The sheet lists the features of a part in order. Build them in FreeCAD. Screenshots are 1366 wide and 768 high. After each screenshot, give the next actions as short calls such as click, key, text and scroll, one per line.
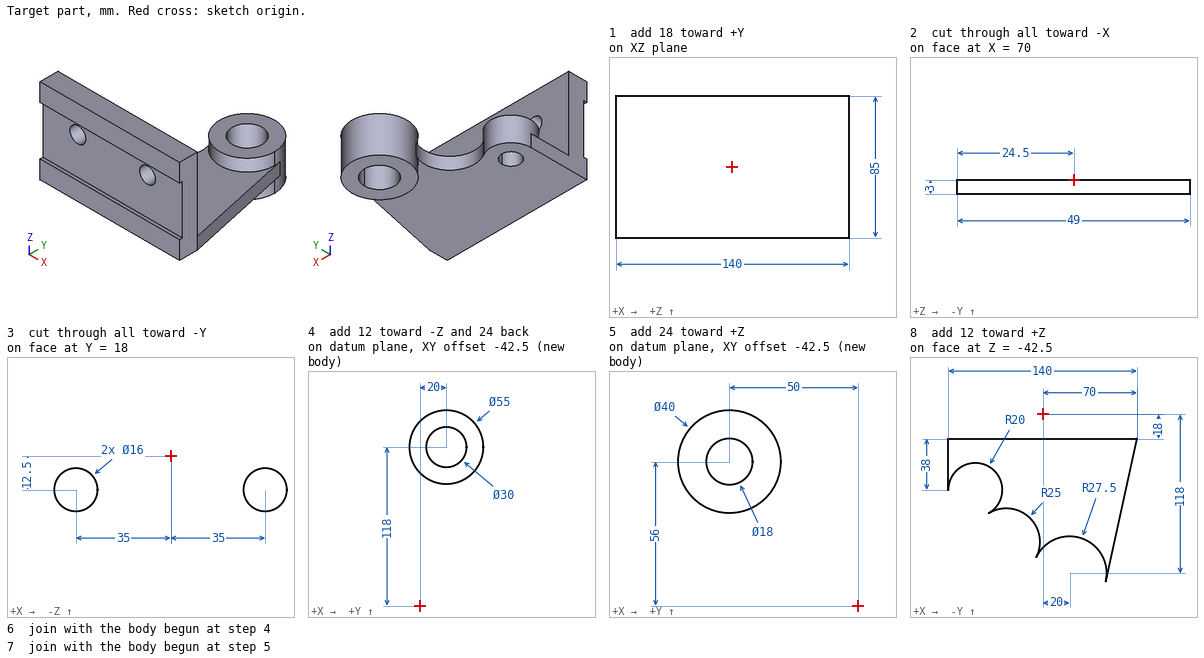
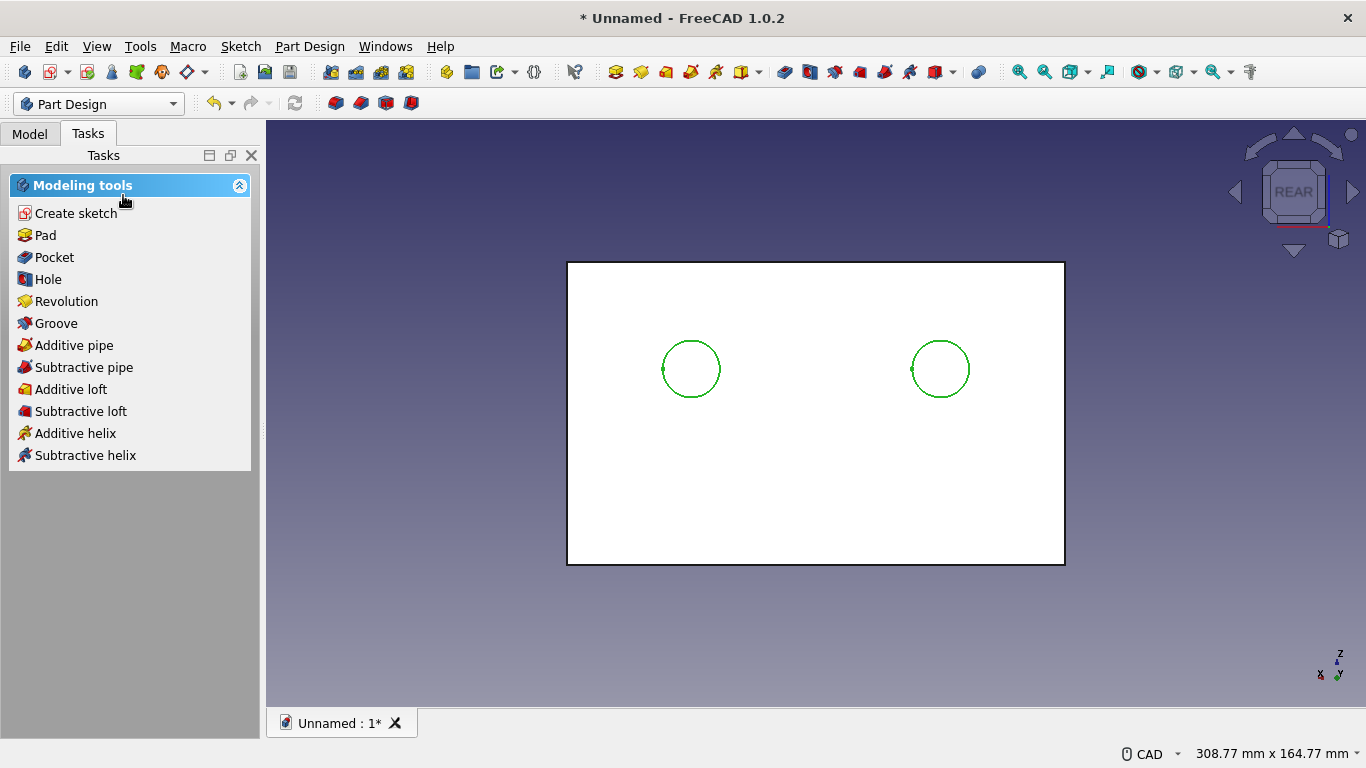
click(785, 72)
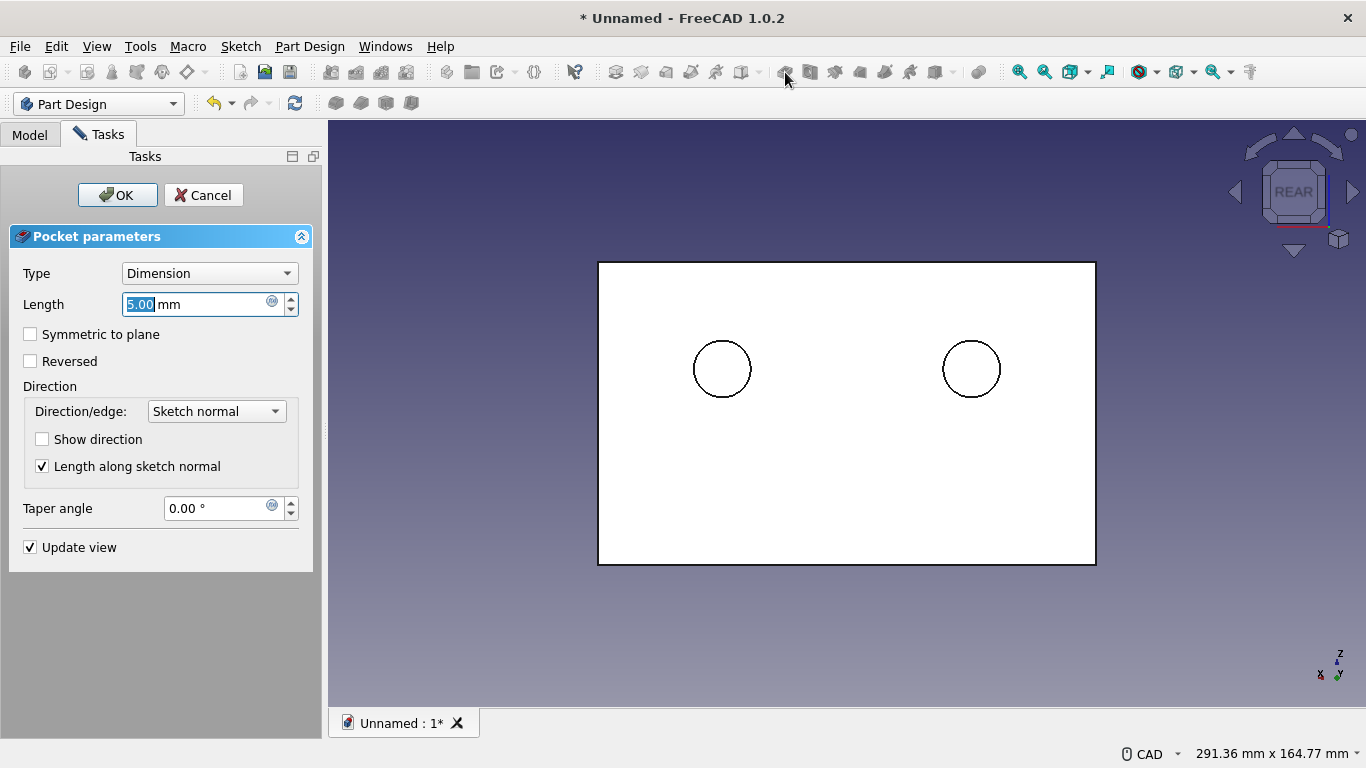
click(210, 274)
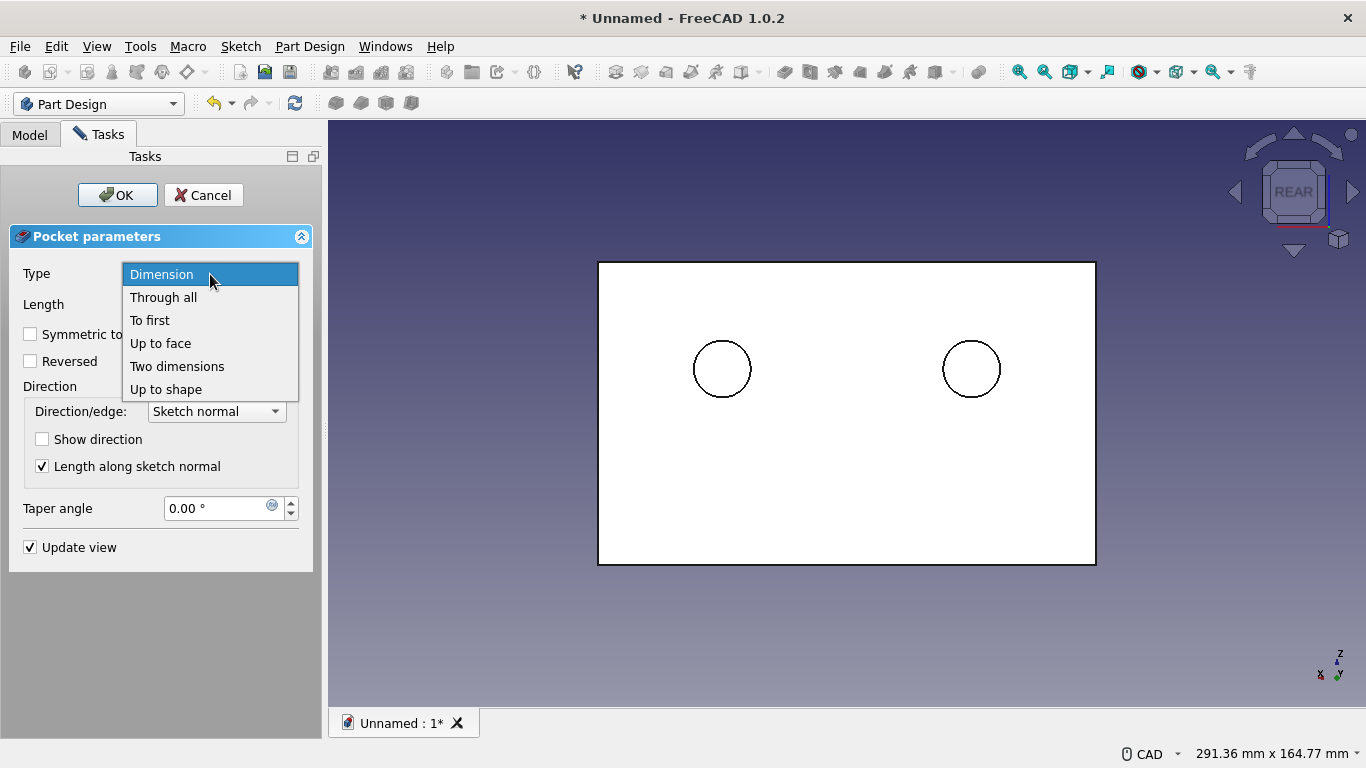
click(208, 298)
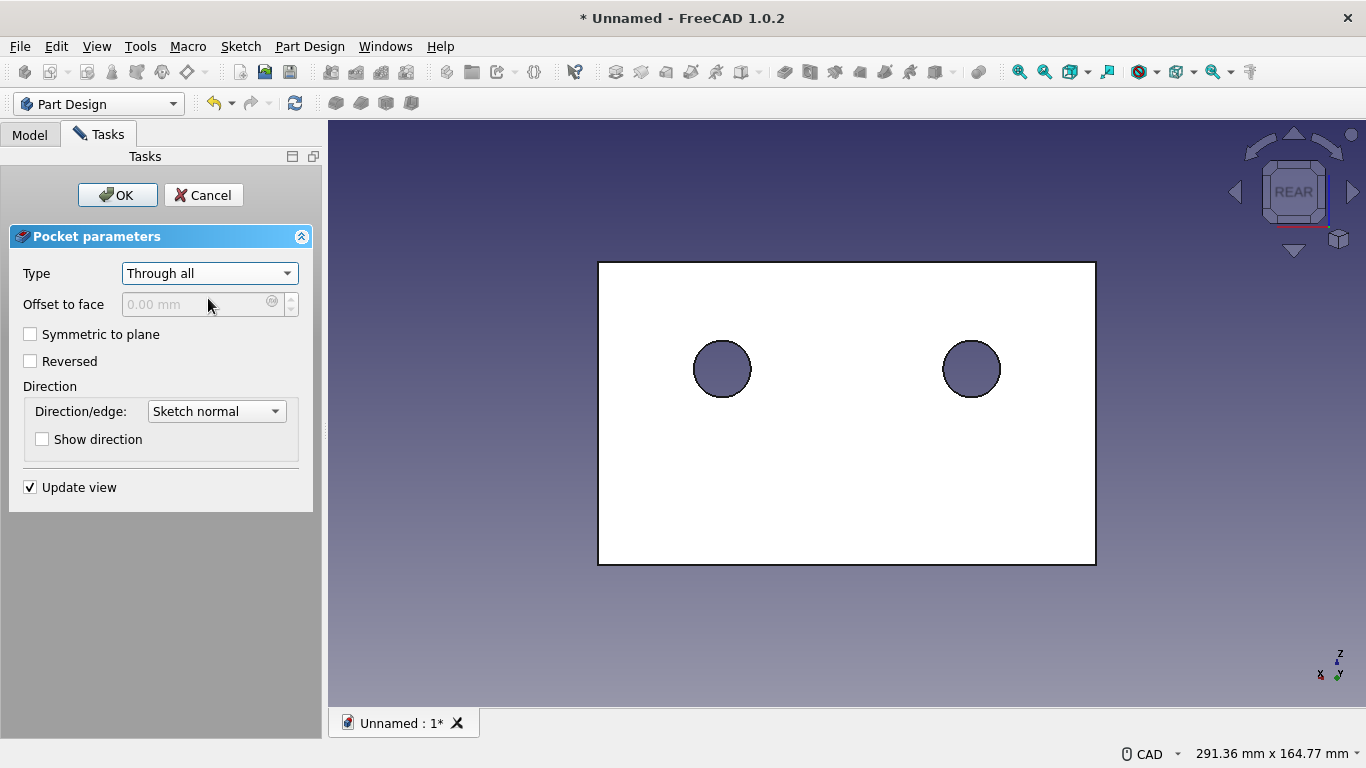
click(118, 195)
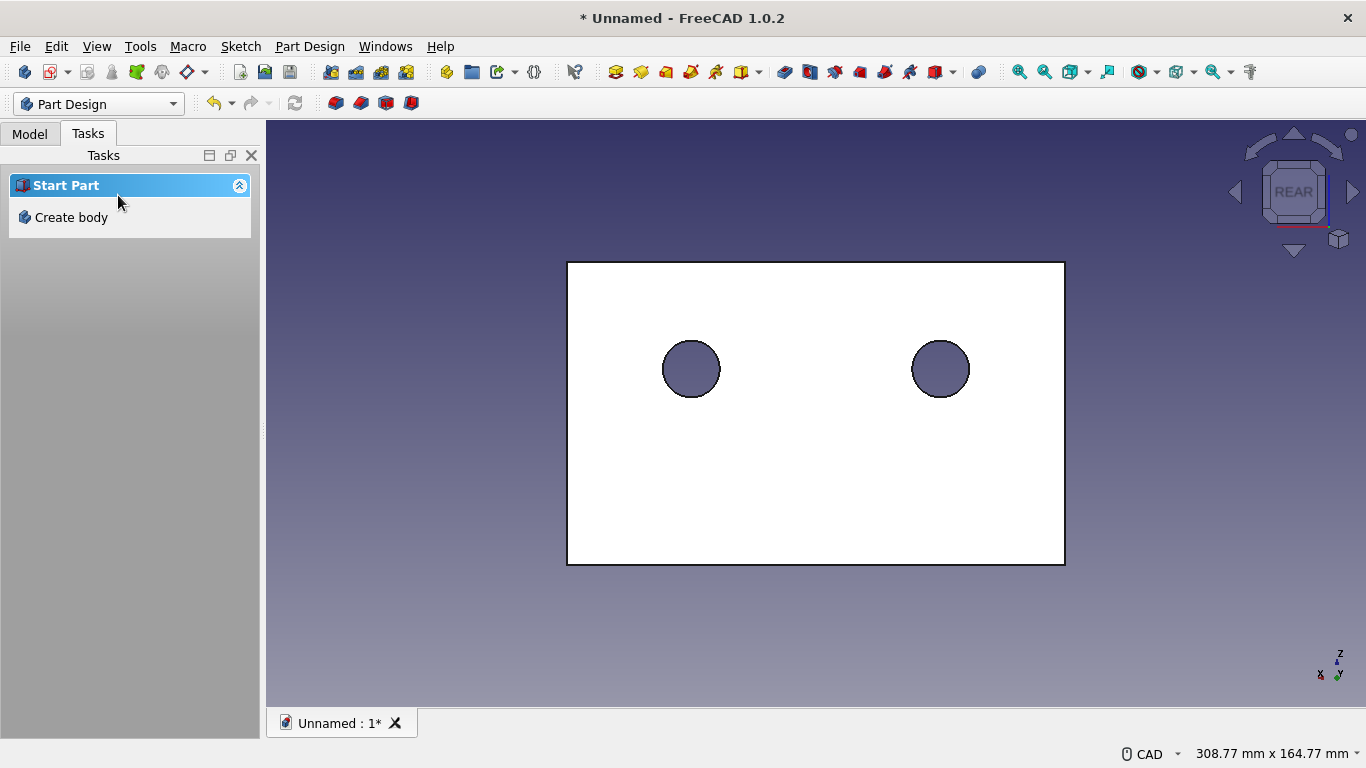
click(25, 72)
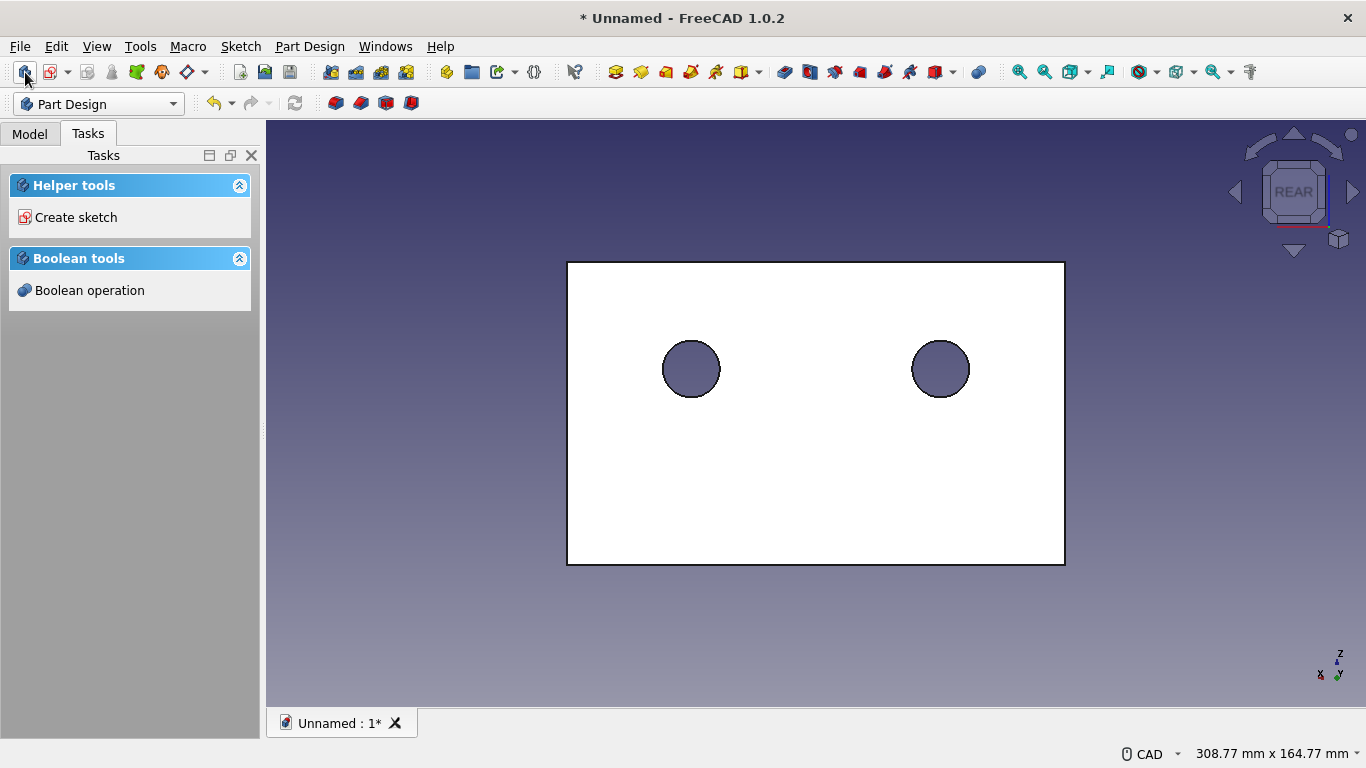
click(30, 134)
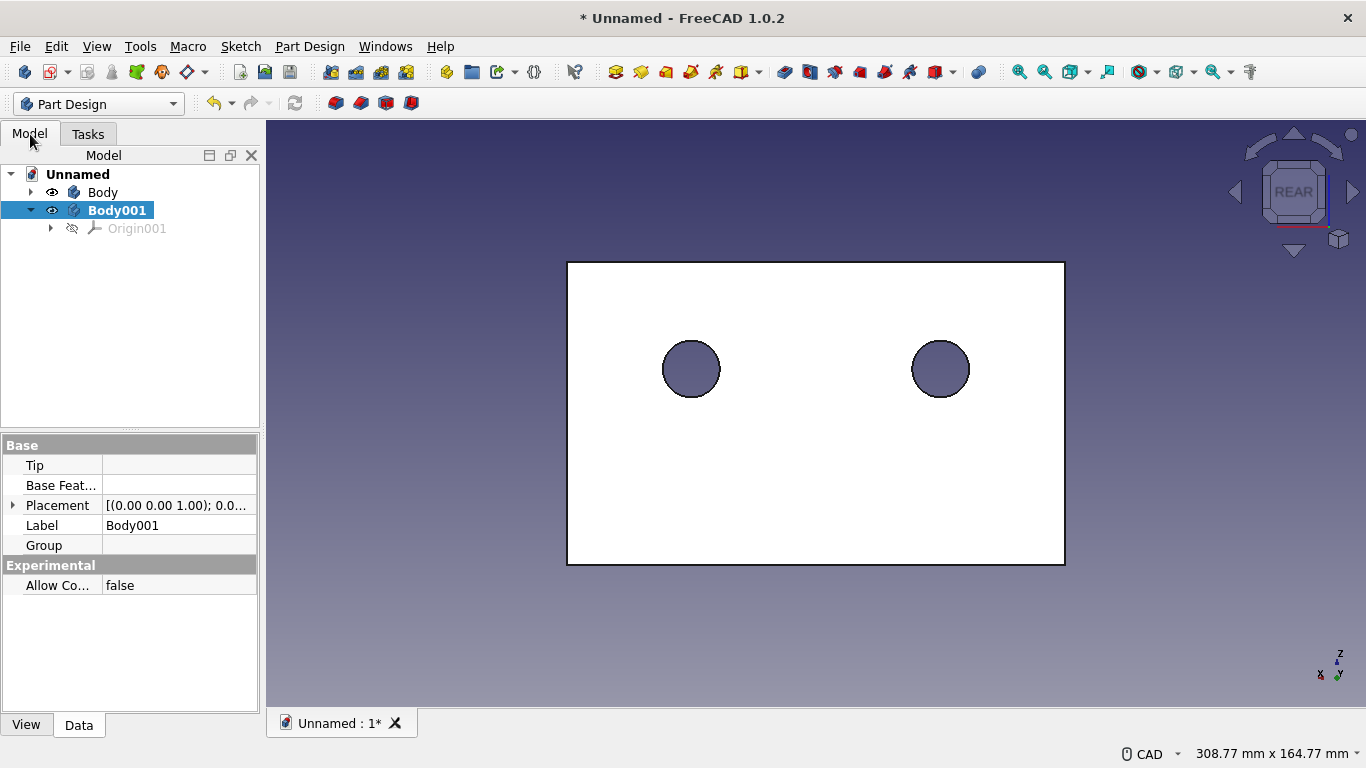
click(51, 228)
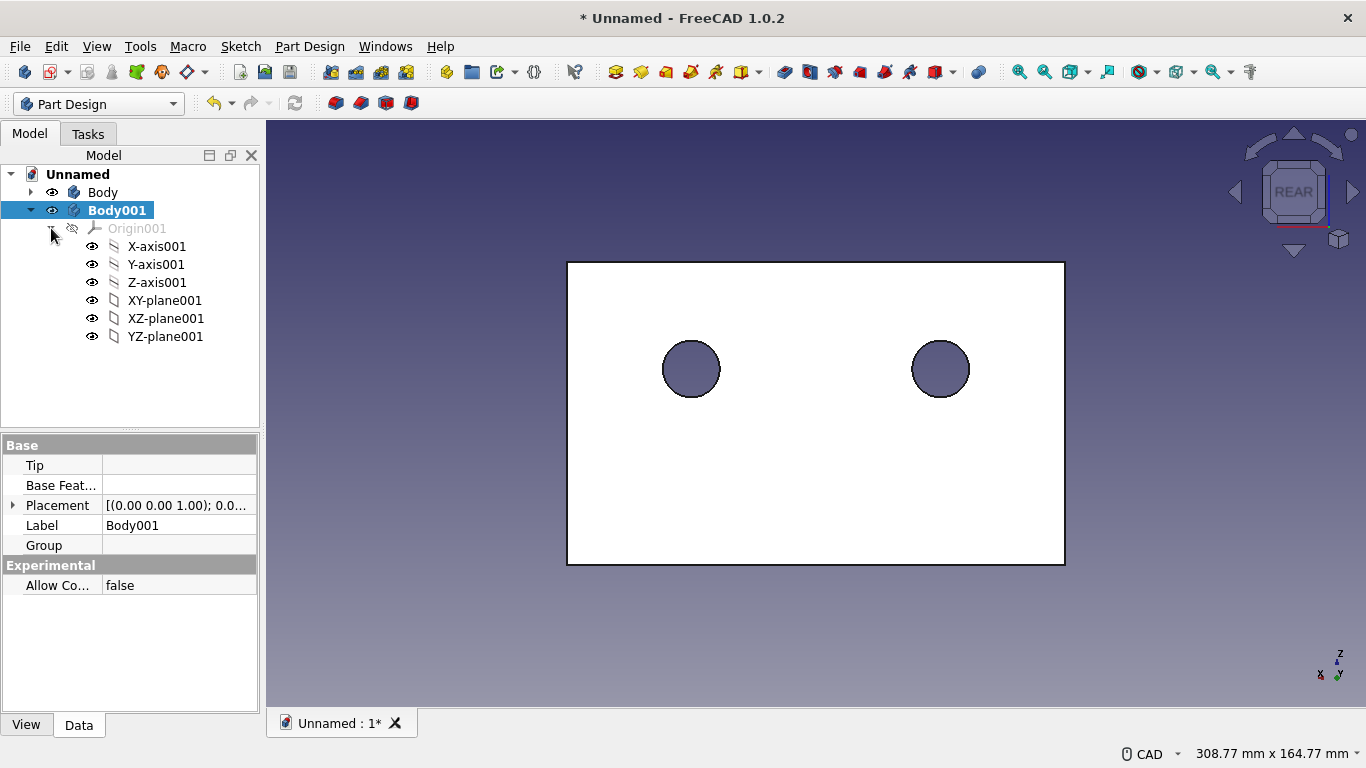
click(137, 300)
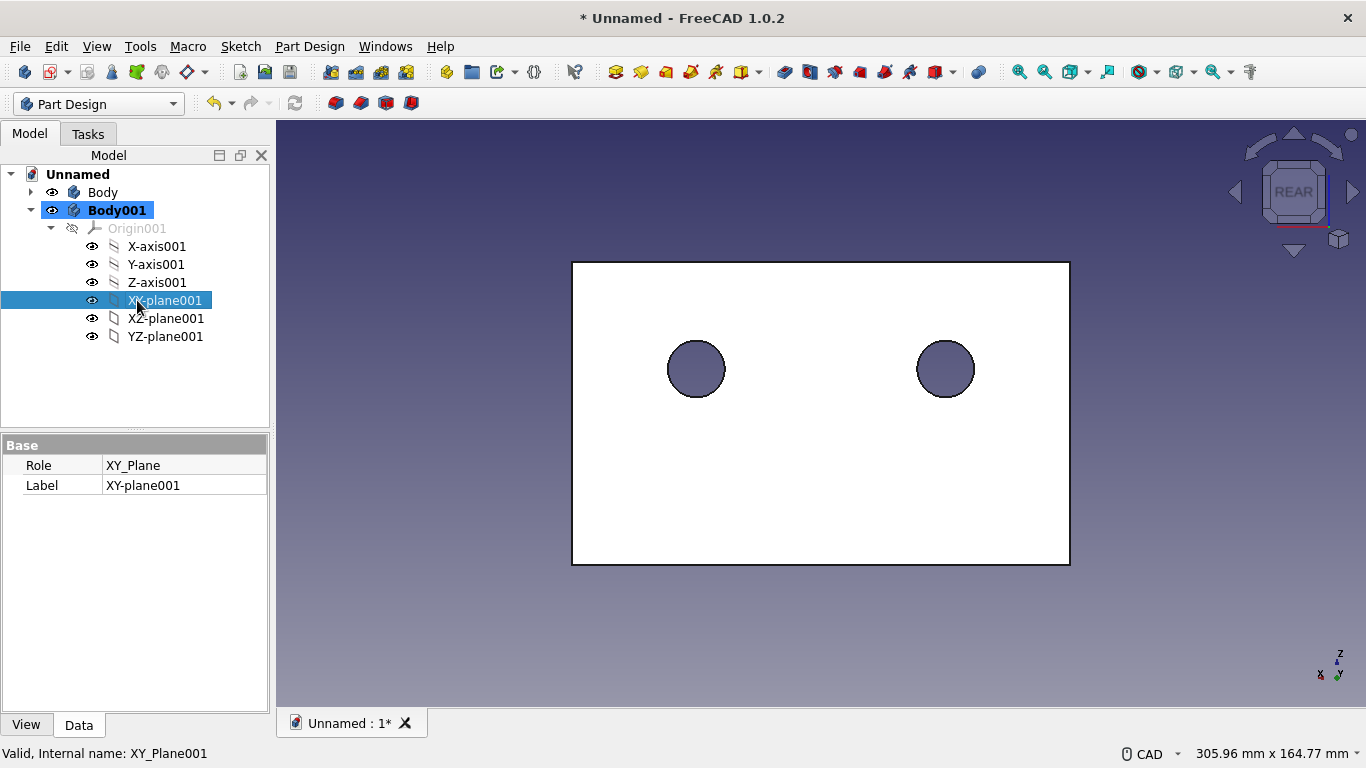
click(186, 72)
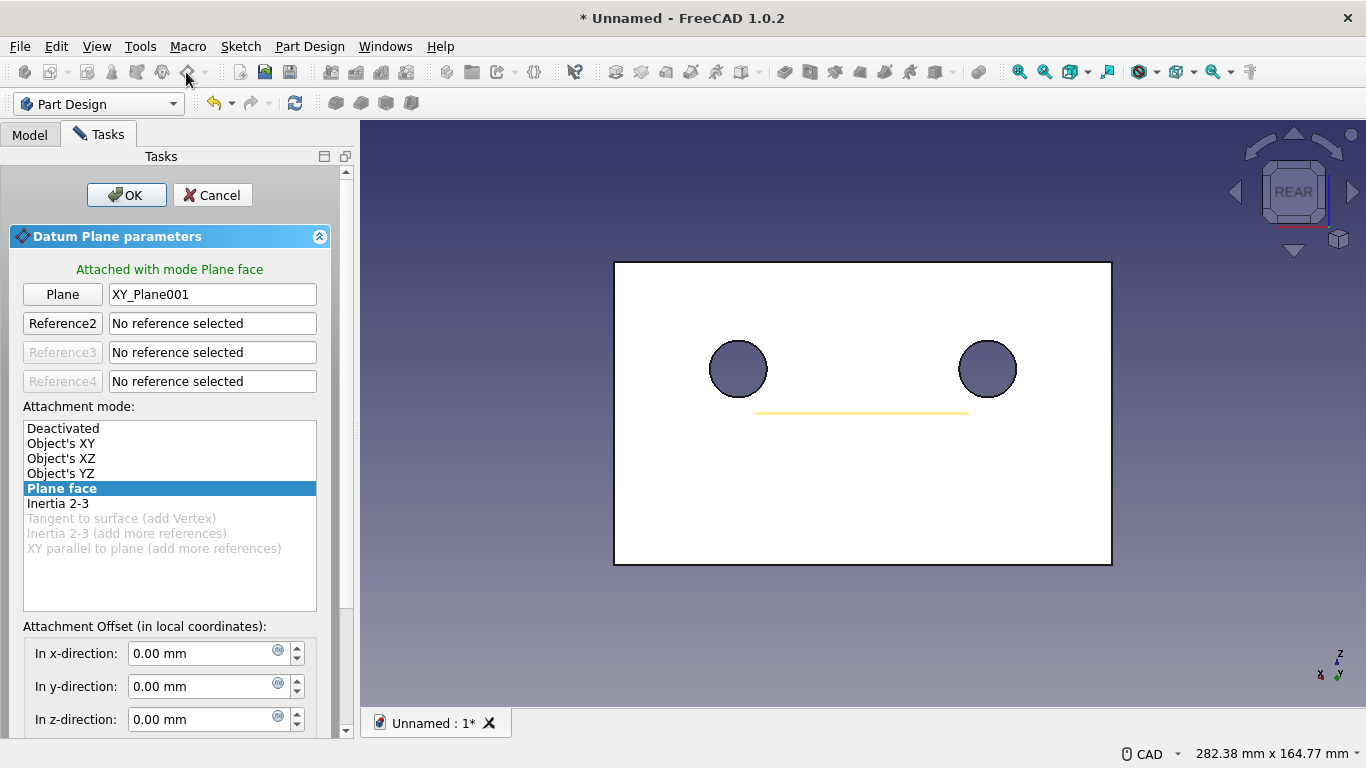
triple_click(210, 720)